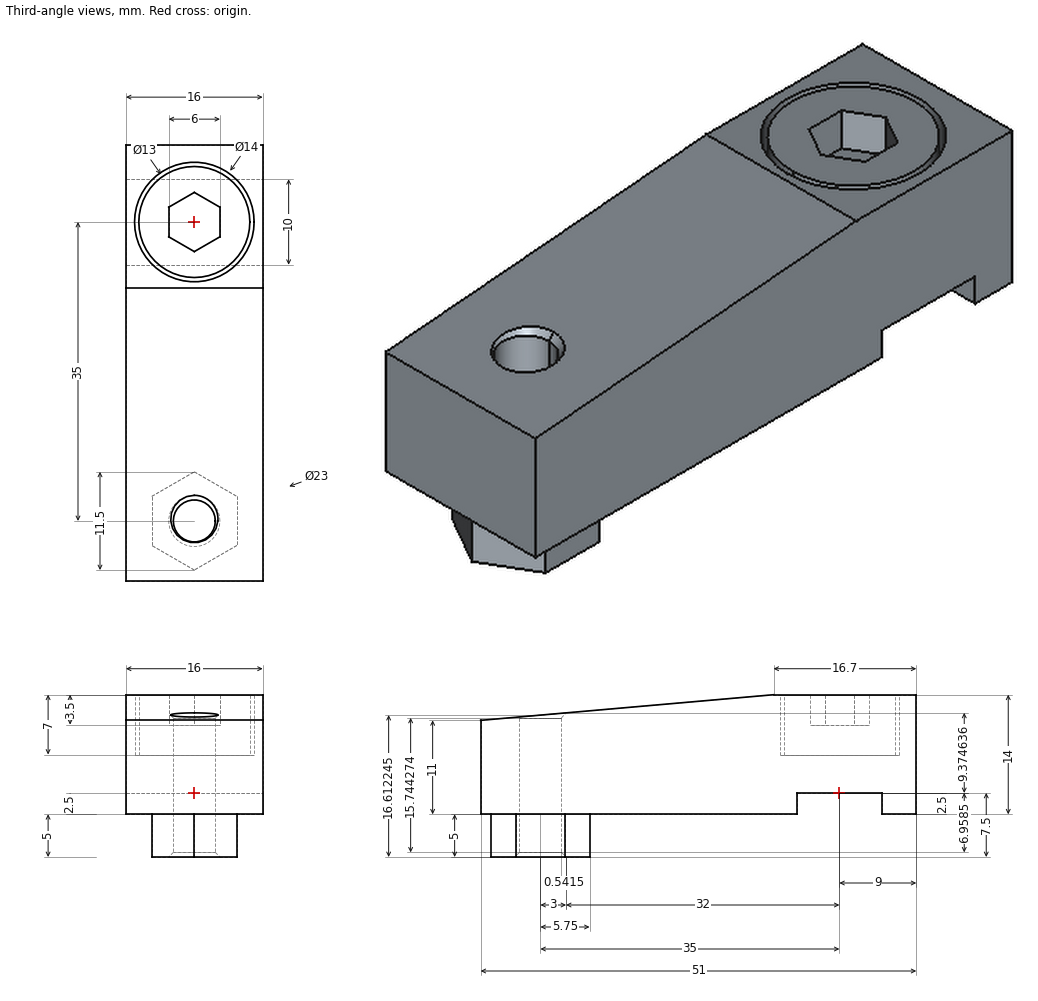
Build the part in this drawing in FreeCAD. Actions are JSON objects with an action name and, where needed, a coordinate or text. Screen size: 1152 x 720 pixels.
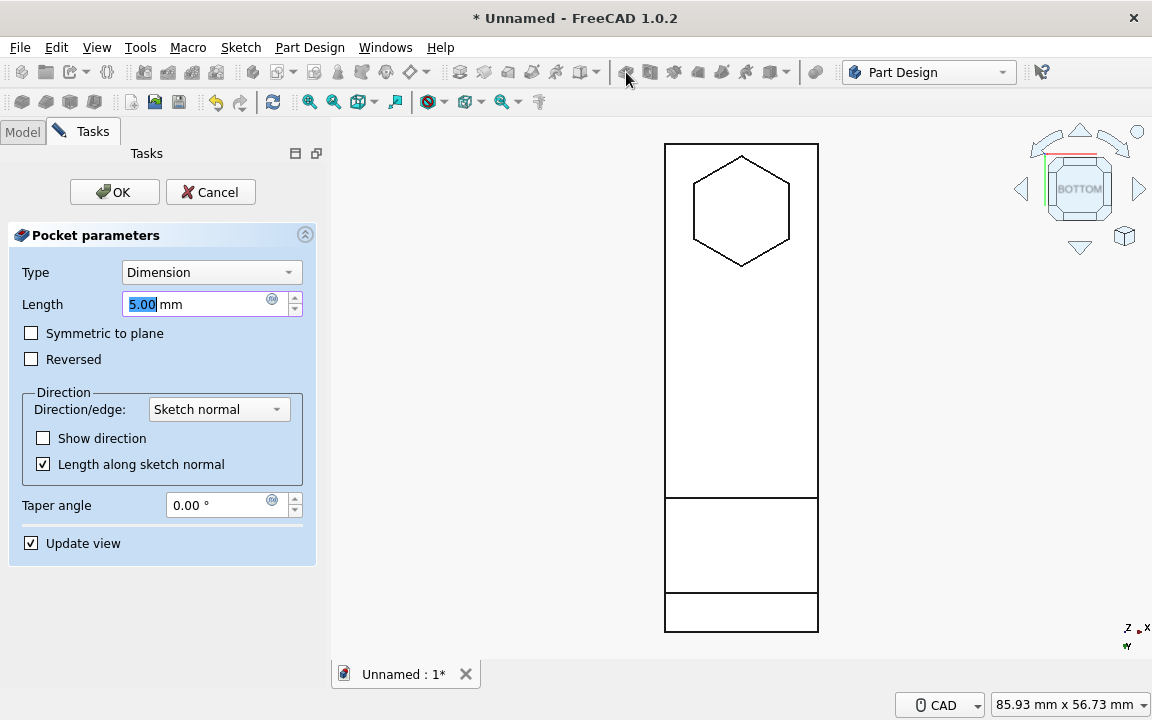
{"action": "type", "text": "5"}
{"action": "key", "text": "Tab"}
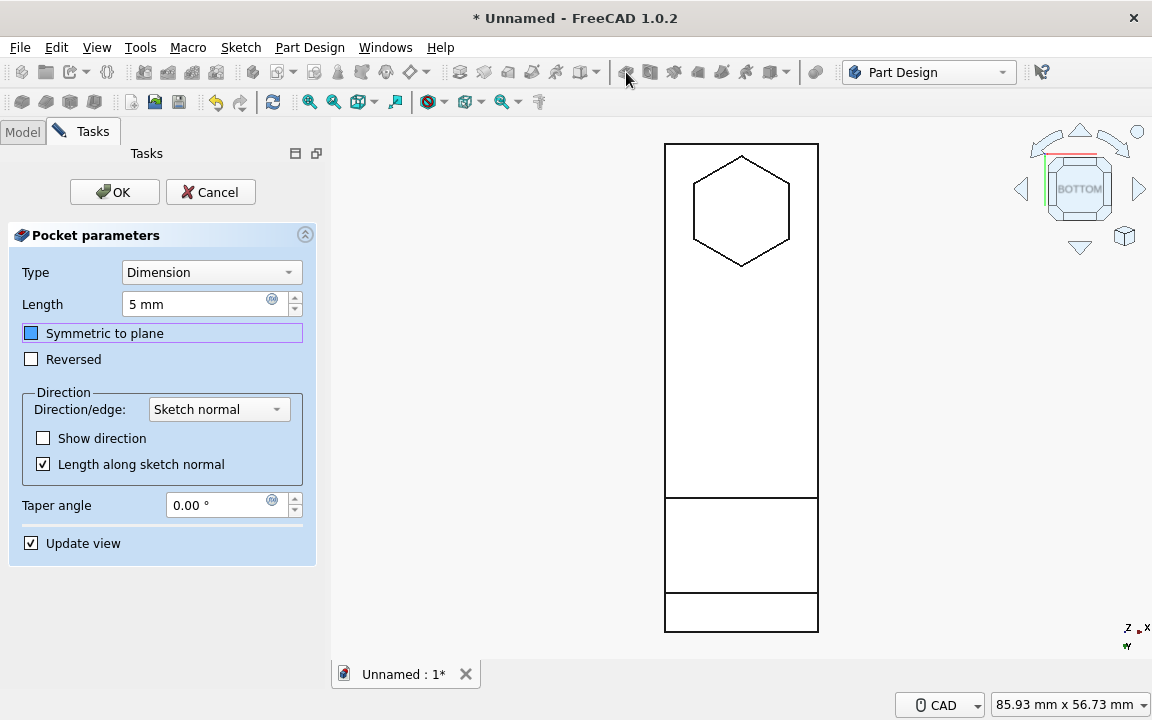
{"action": "left_click", "coordinate": [115, 192]}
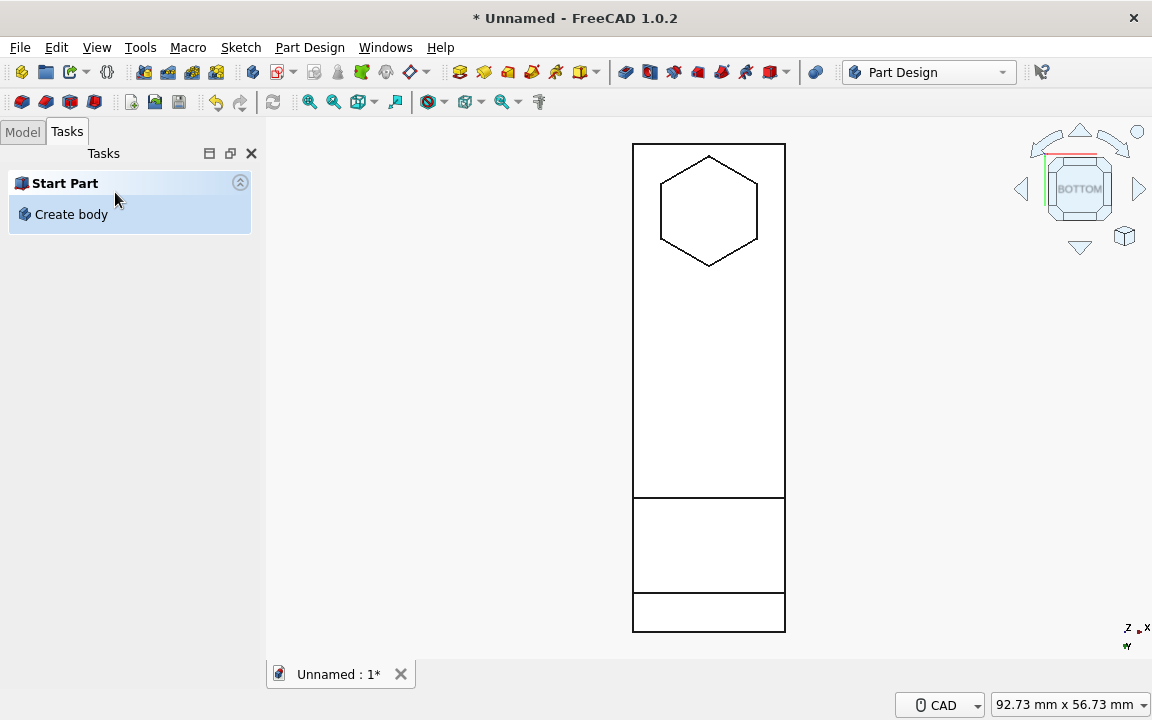
{"action": "left_click", "coordinate": [278, 72]}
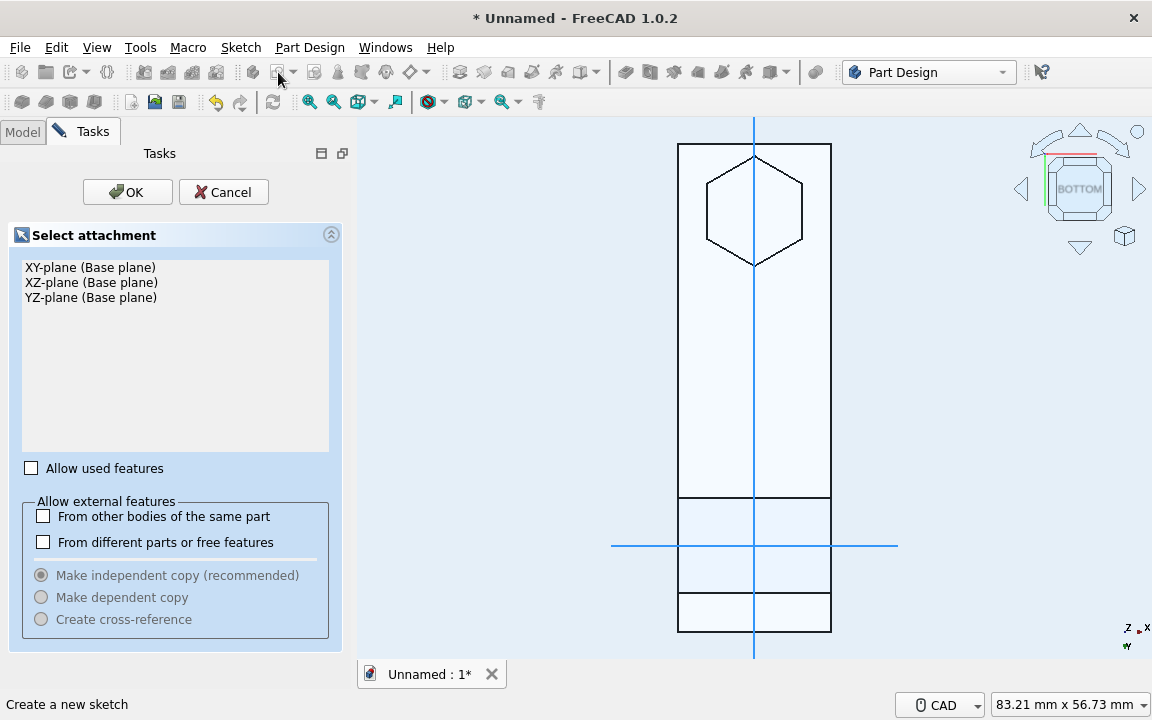
{"action": "left_click", "coordinate": [82, 298]}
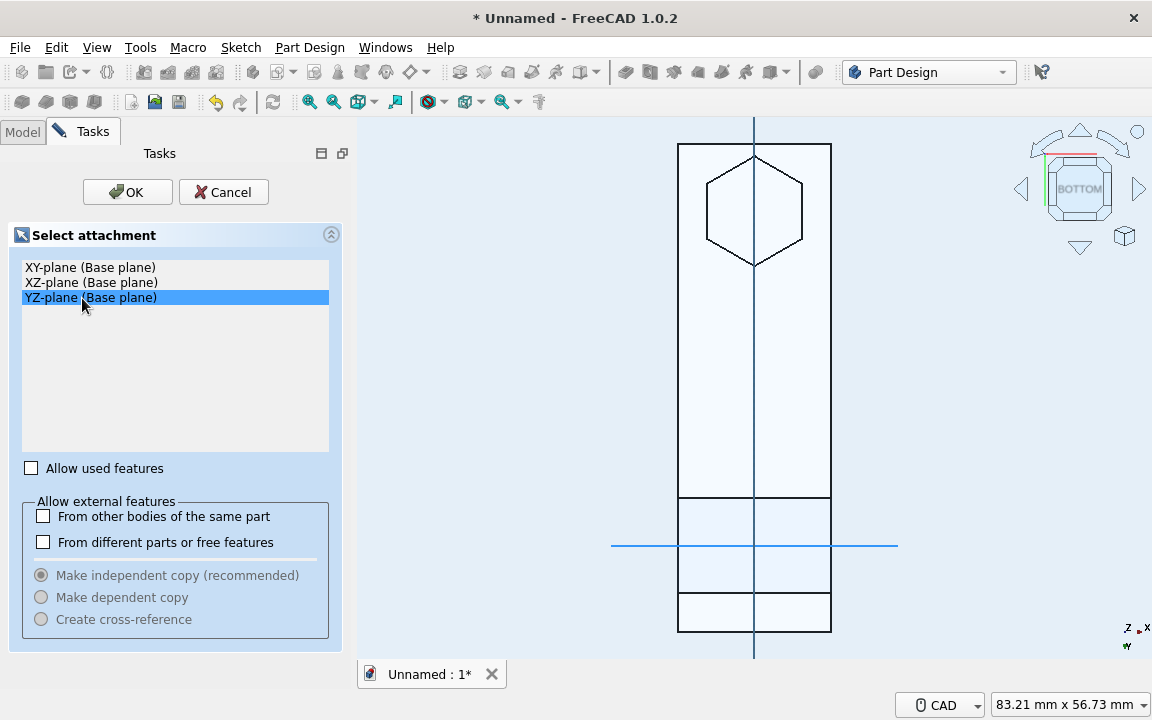
{"action": "left_click", "coordinate": [128, 192]}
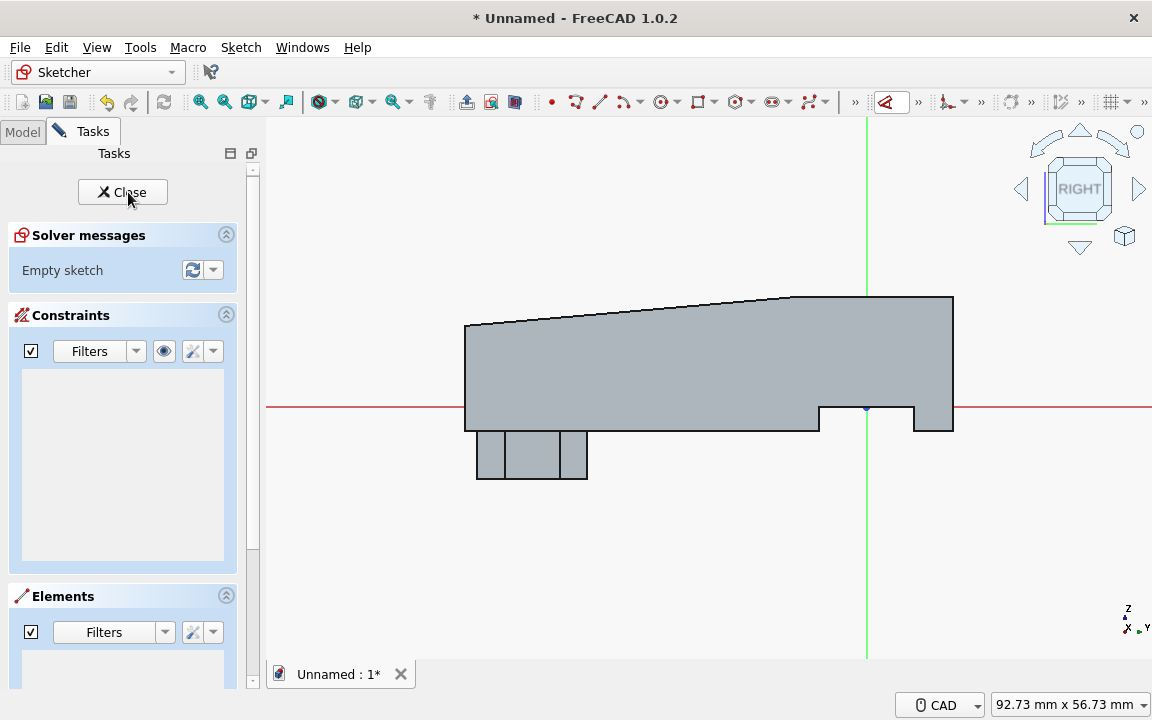
{"action": "left_click", "coordinate": [516, 102]}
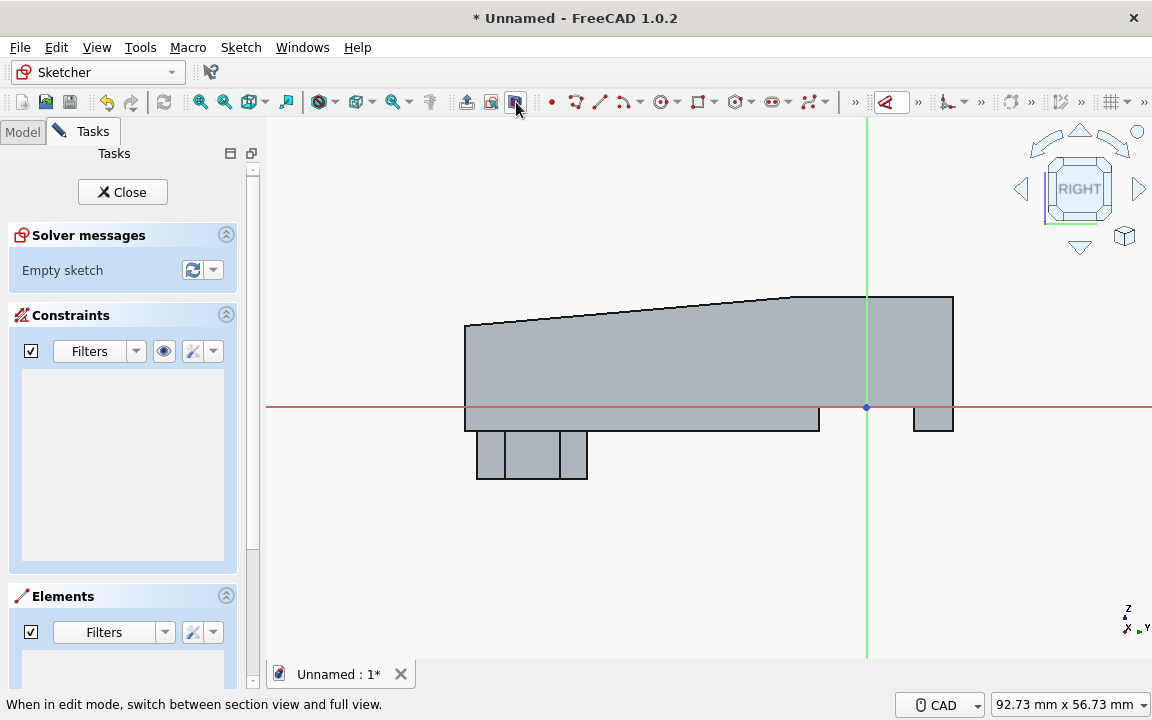
{"action": "scroll", "coordinate": [819, 321], "scroll_direction": "up", "scroll_amount": 2}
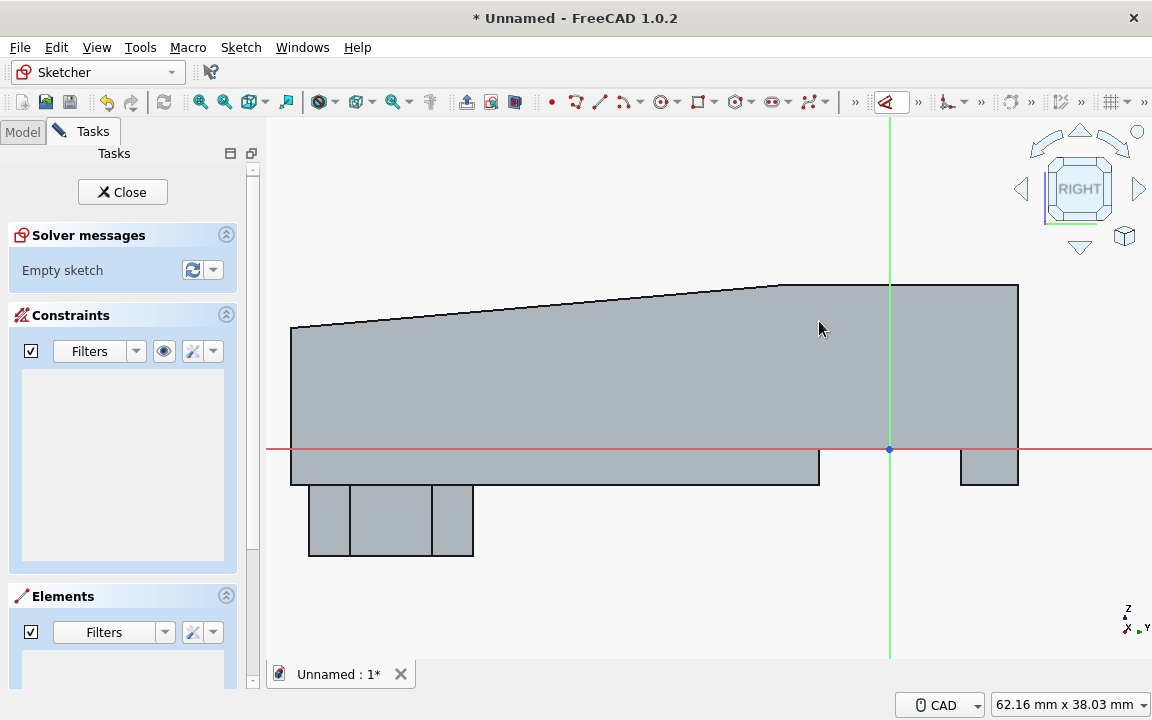
{"action": "key", "text": "g m"}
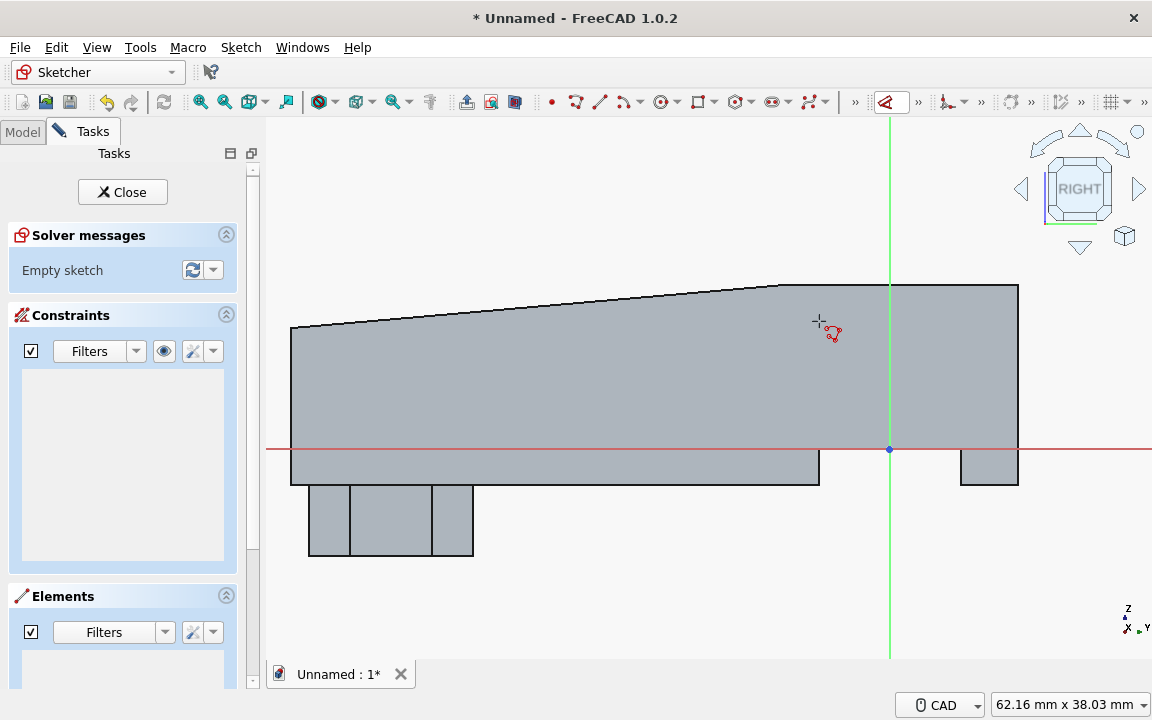
{"action": "left_click", "coordinate": [434, 556]}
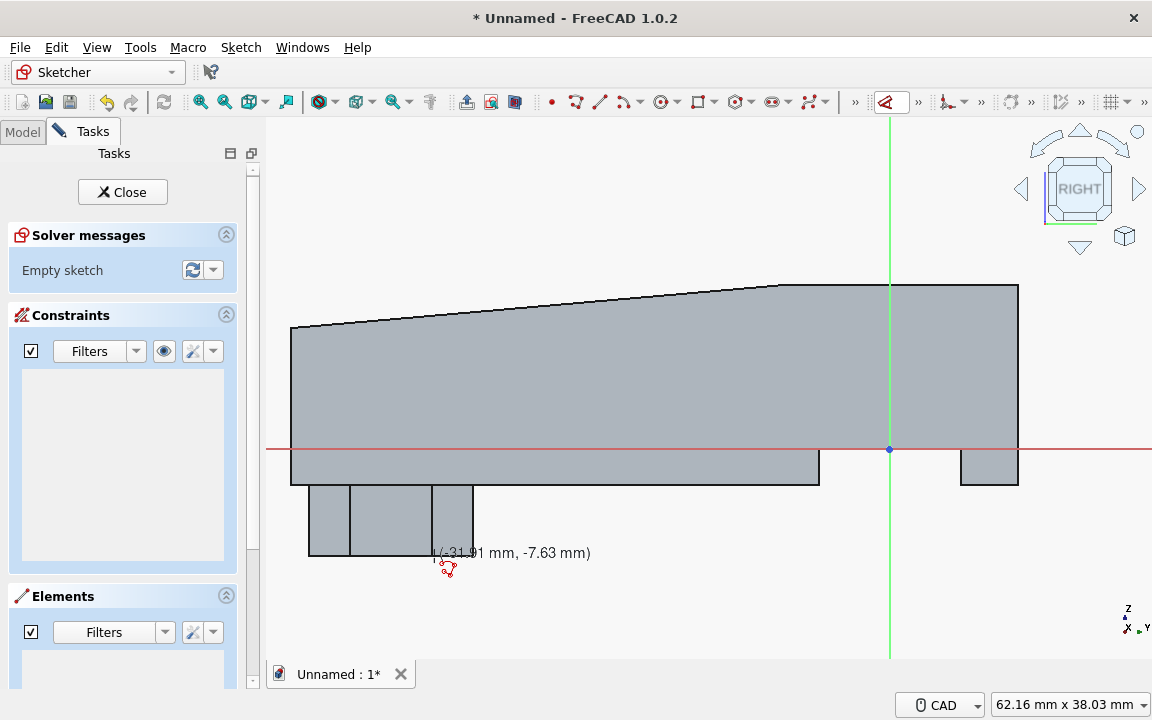
{"action": "scroll", "coordinate": [426, 548], "scroll_direction": "up", "scroll_amount": 2}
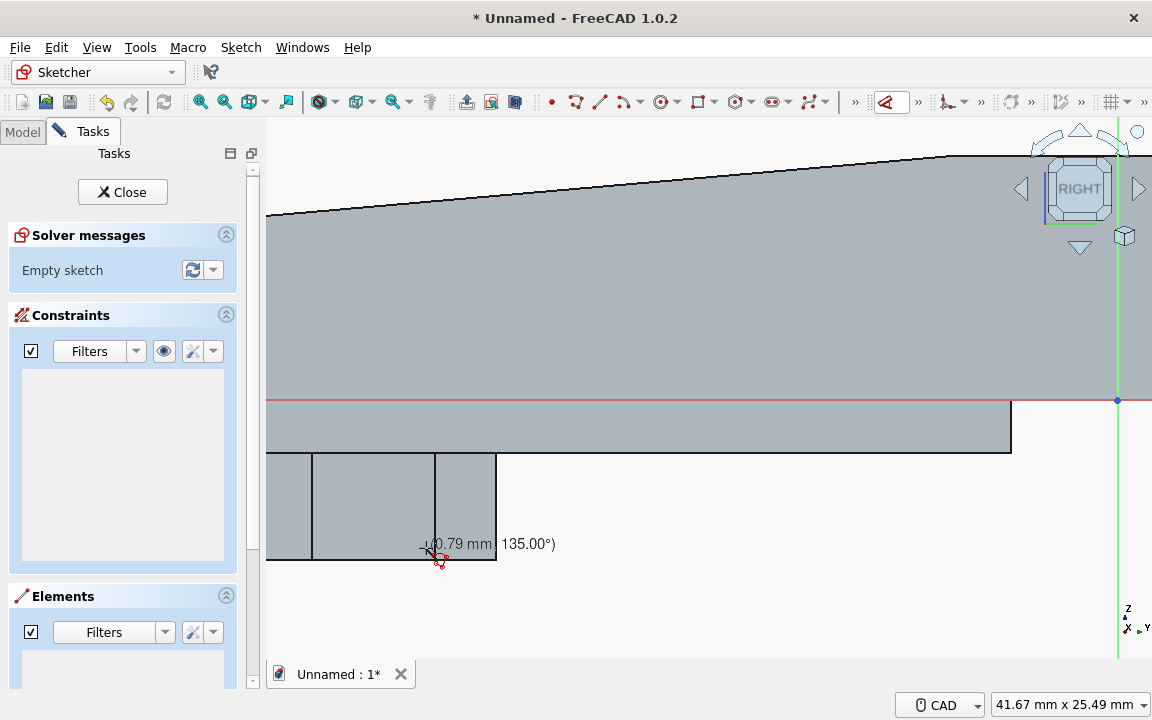
{"action": "left_click", "coordinate": [426, 548]}
{"action": "left_click", "coordinate": [426, 214]}
{"action": "left_click", "coordinate": [437, 201]}
{"action": "left_click", "coordinate": [374, 207]}
{"action": "left_click", "coordinate": [374, 560]}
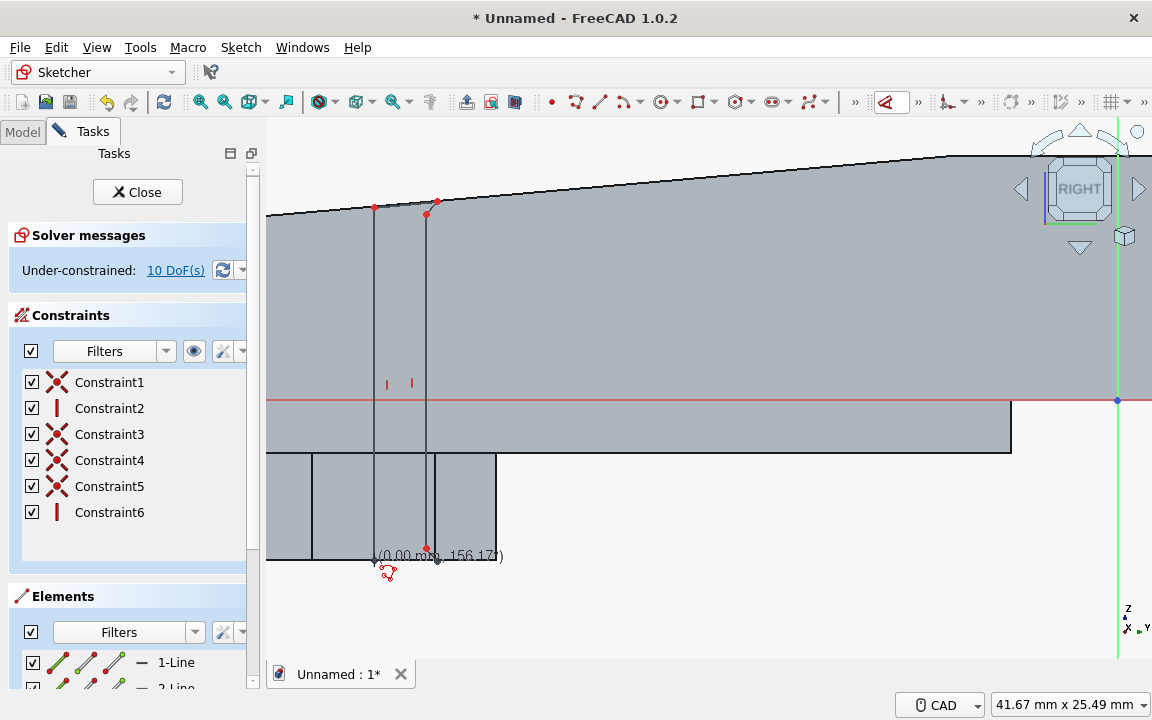
{"action": "scroll", "coordinate": [437, 560], "scroll_direction": "up", "scroll_amount": 4}